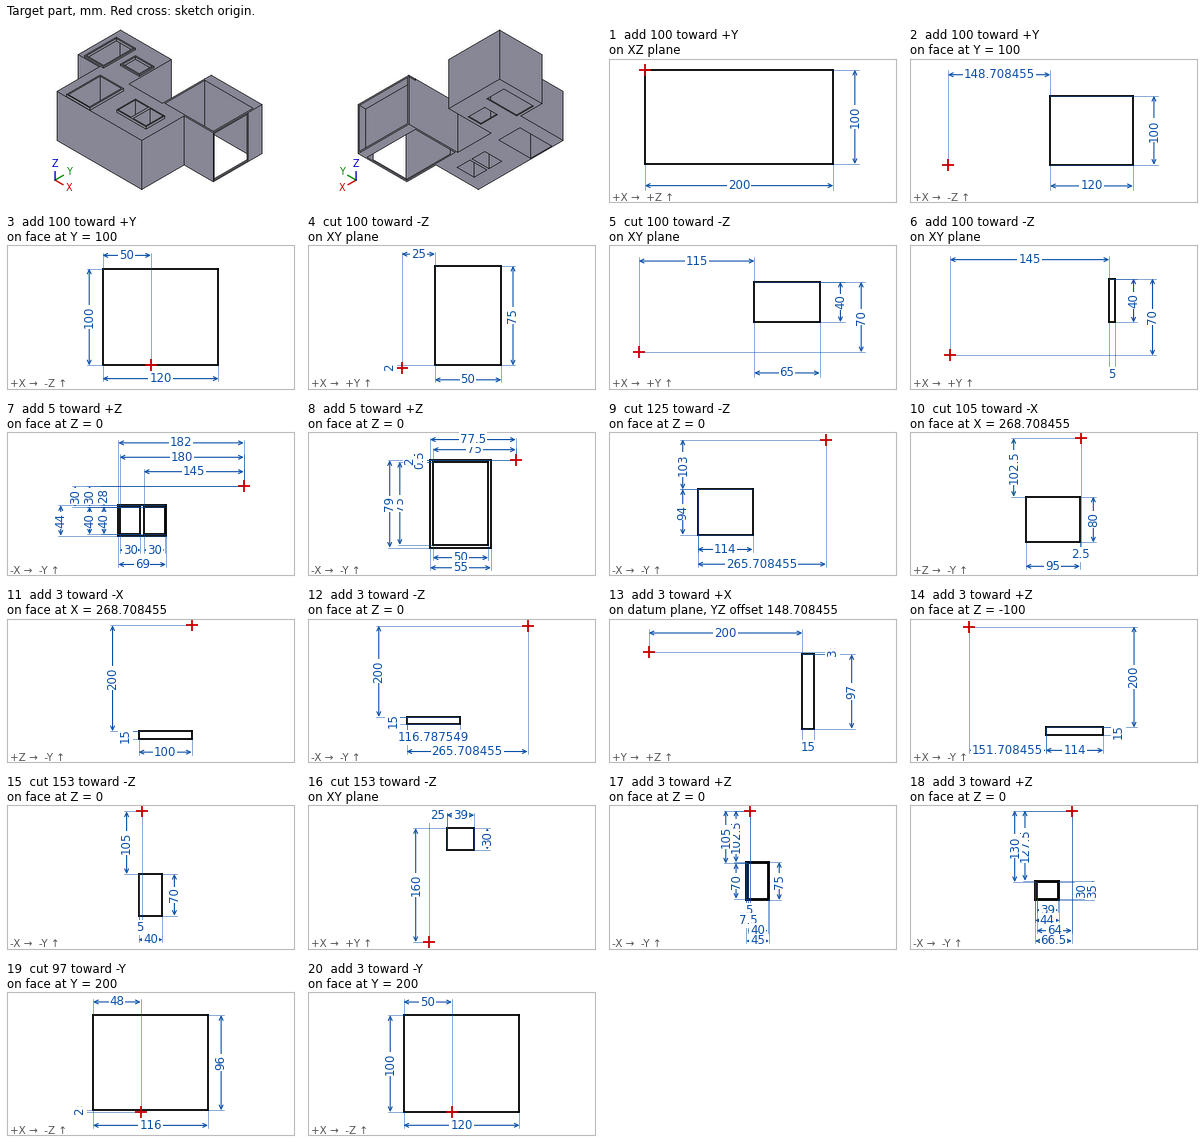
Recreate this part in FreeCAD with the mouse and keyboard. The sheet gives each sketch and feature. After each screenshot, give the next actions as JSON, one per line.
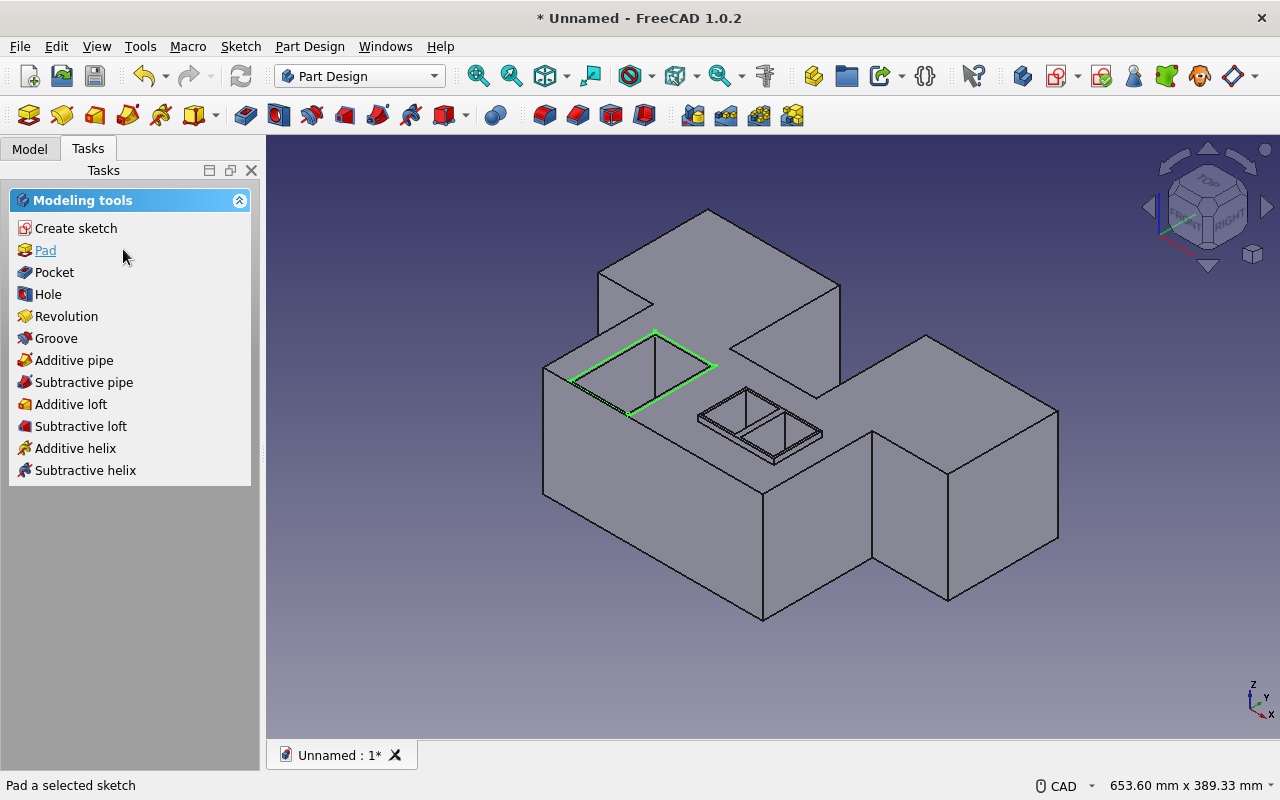
{"action": "left_click", "coordinate": [29, 116]}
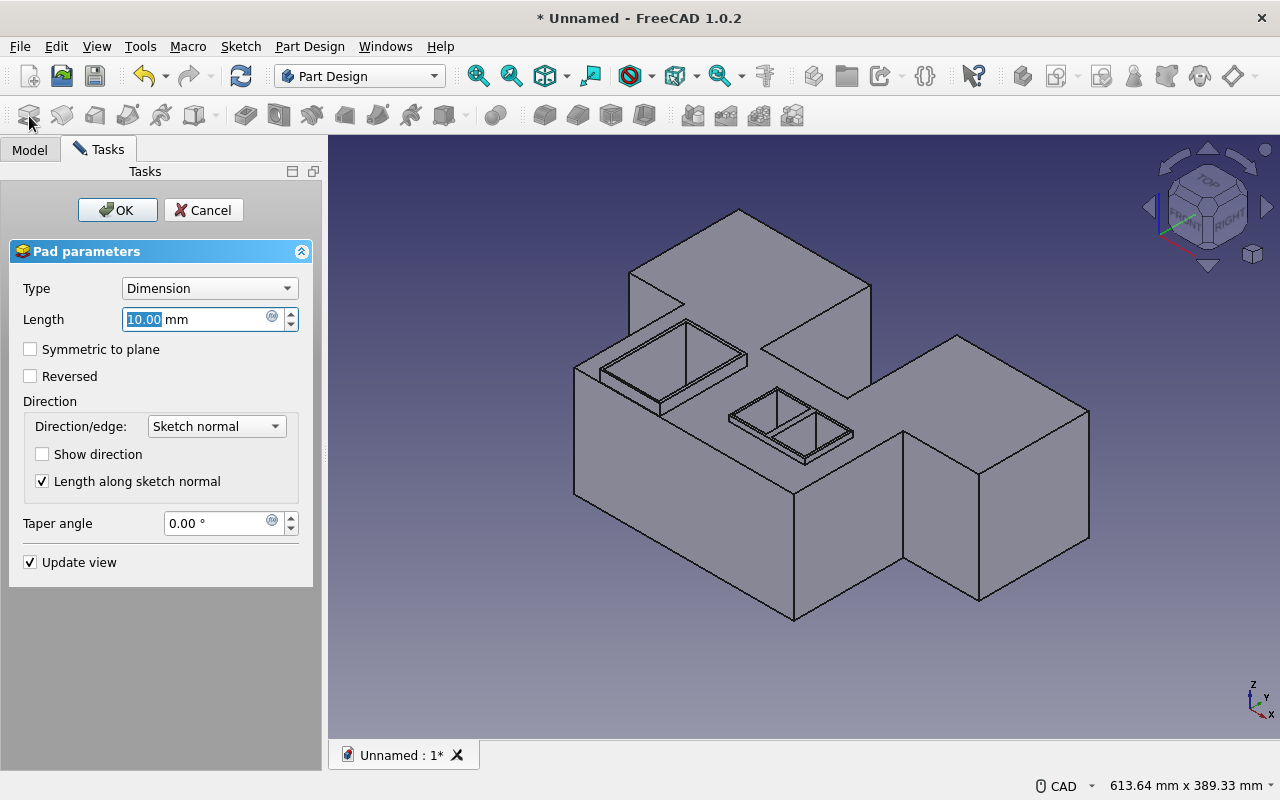
{"action": "type", "text": "5"}
{"action": "key", "text": "Tab"}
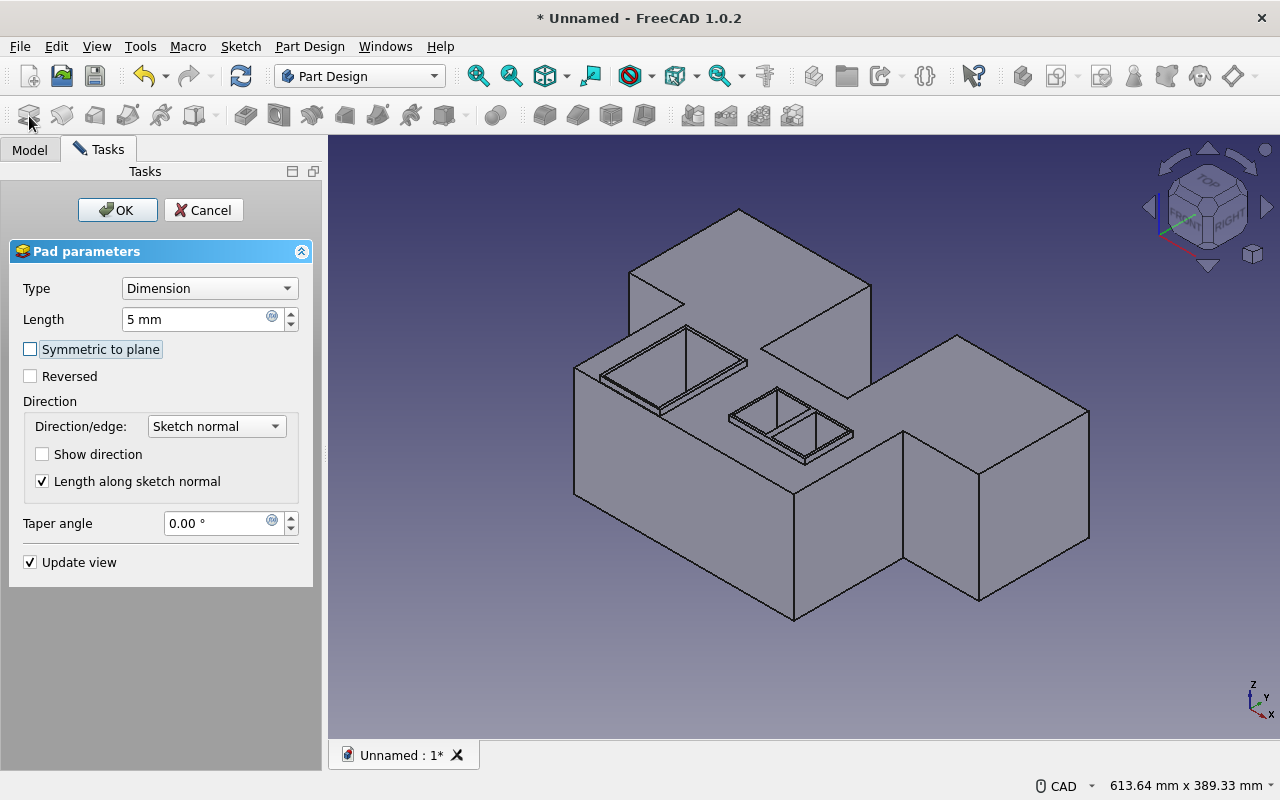
{"action": "left_click", "coordinate": [118, 210]}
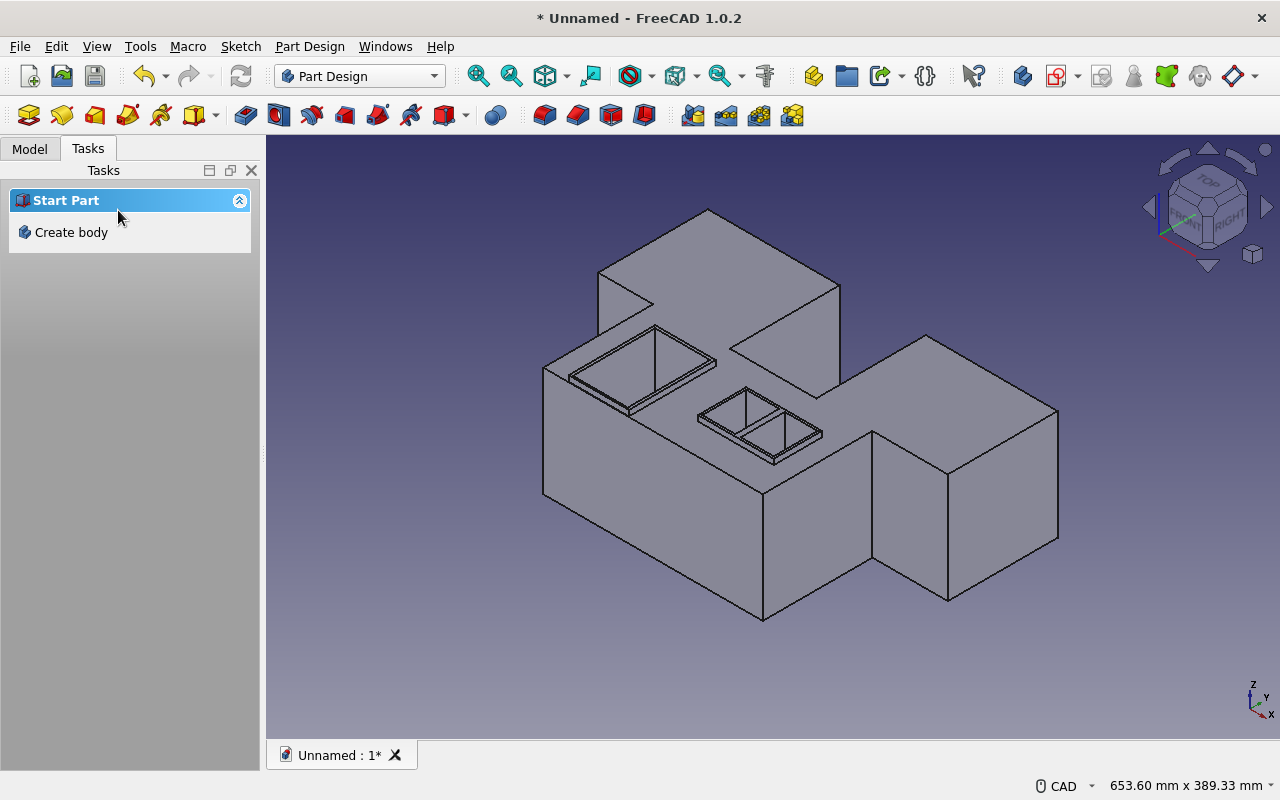
{"action": "left_click", "coordinate": [936, 394]}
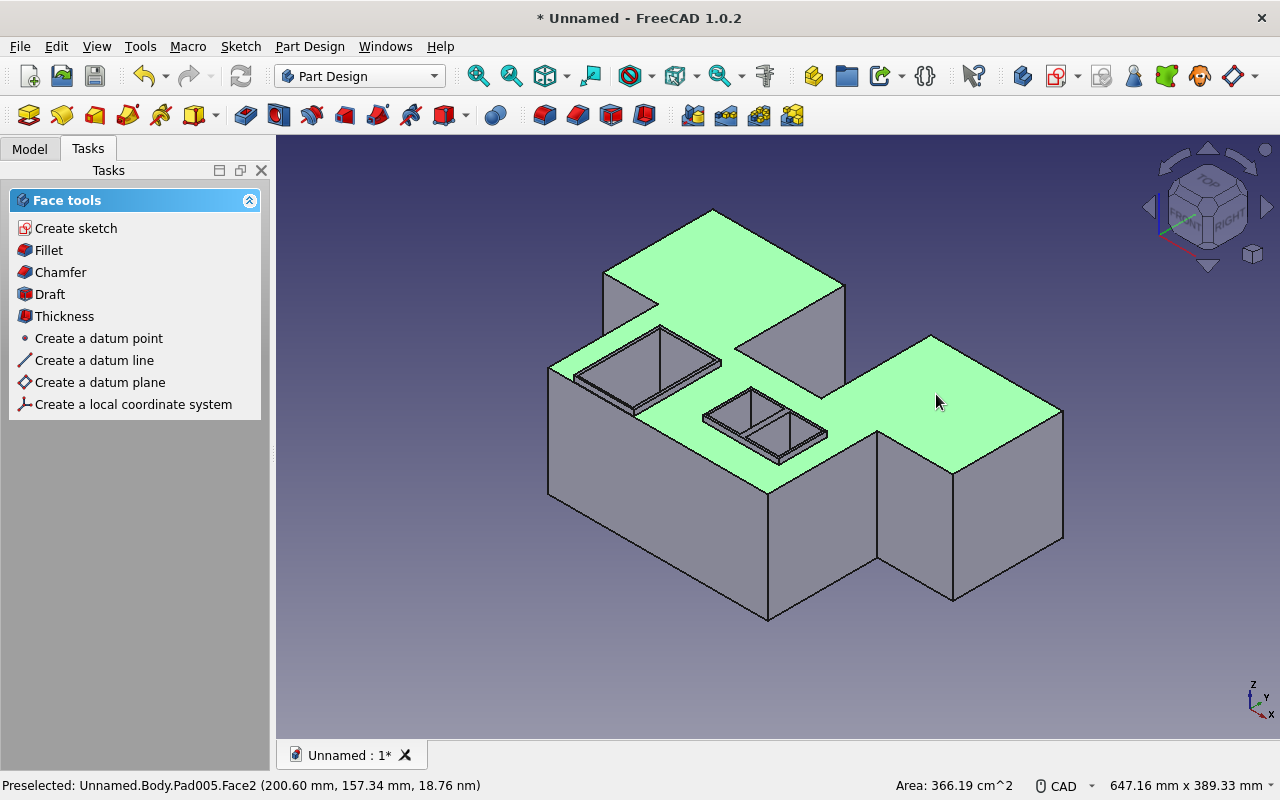
{"action": "left_click", "coordinate": [1056, 76]}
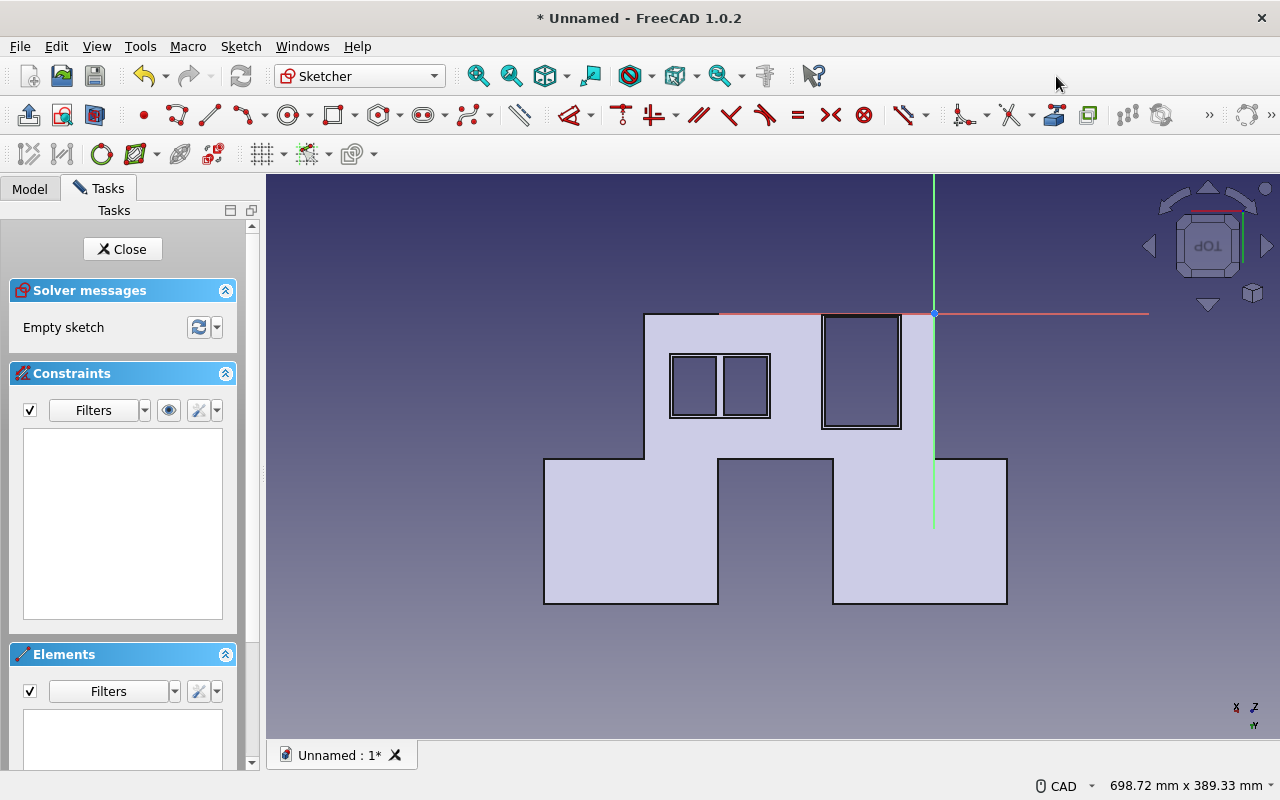
{"action": "left_click", "coordinate": [332, 116]}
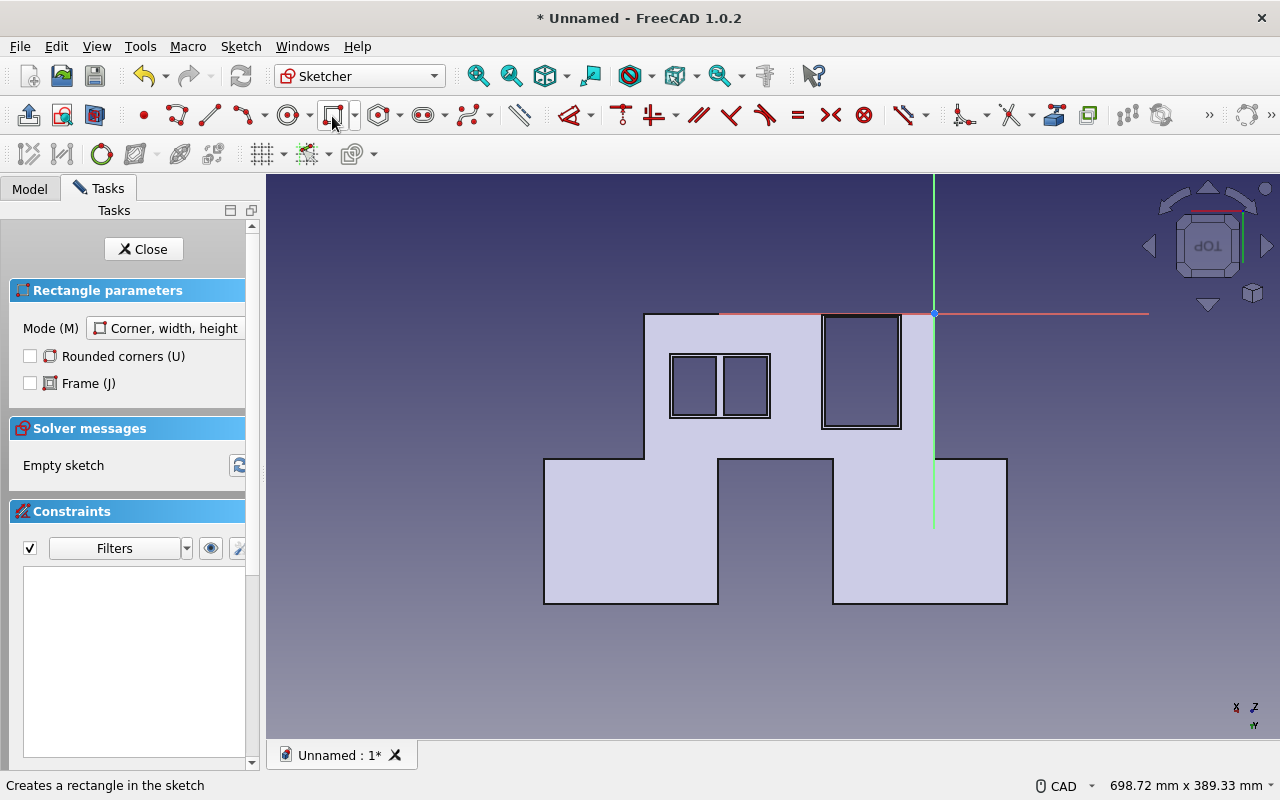
{"action": "left_click", "coordinate": [549, 463]}
{"action": "mouse_move", "coordinate": [714, 600]}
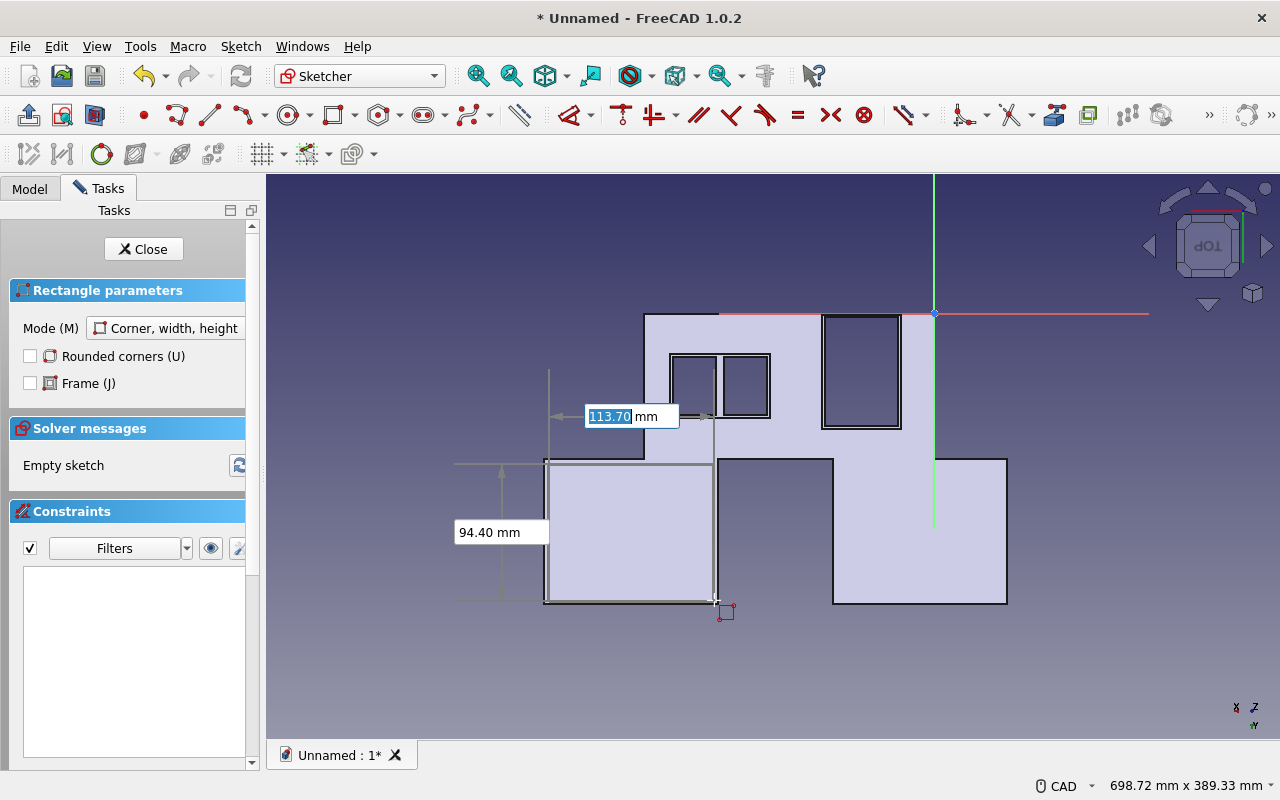
{"action": "type", "text": "114"}
{"action": "key", "text": "Tab"}
{"action": "type", "text": "94"}
{"action": "key", "text": "Return"}
{"action": "key", "text": "Escape"}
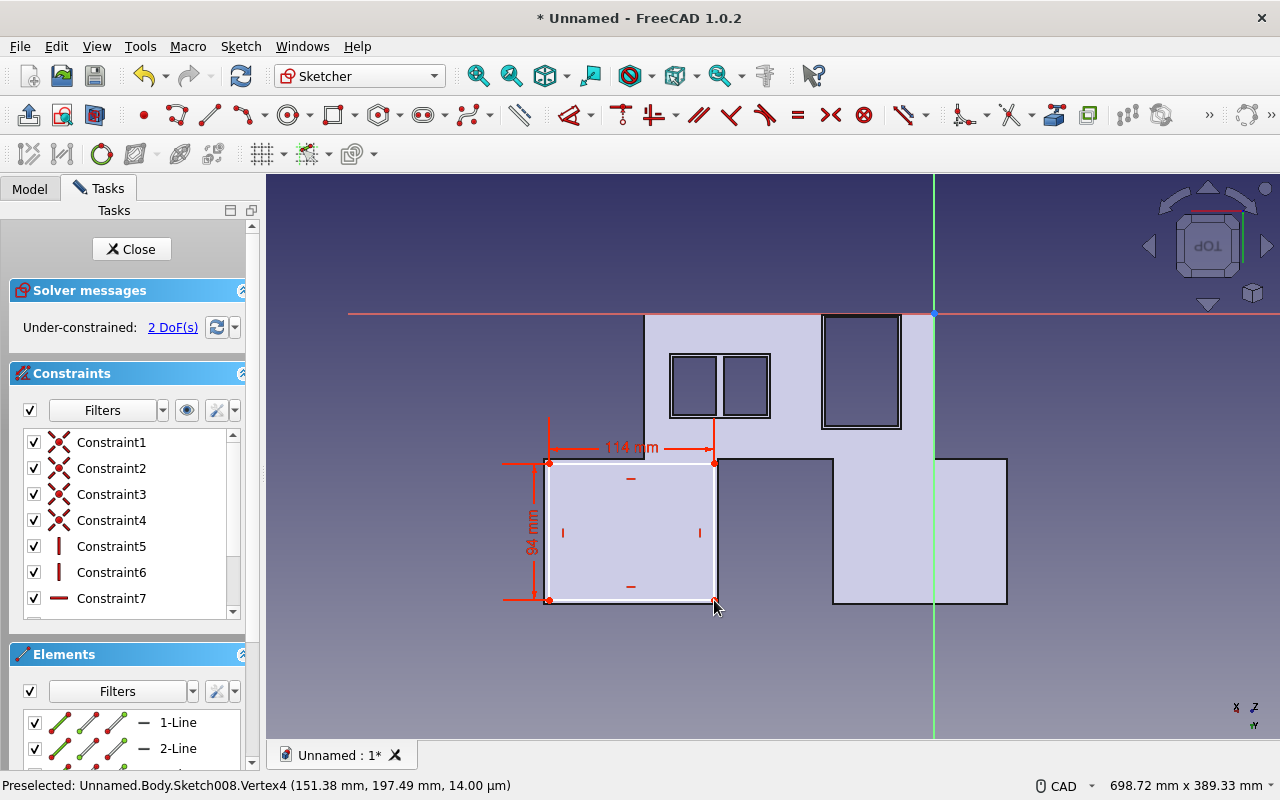
{"action": "left_click", "coordinate": [568, 116]}